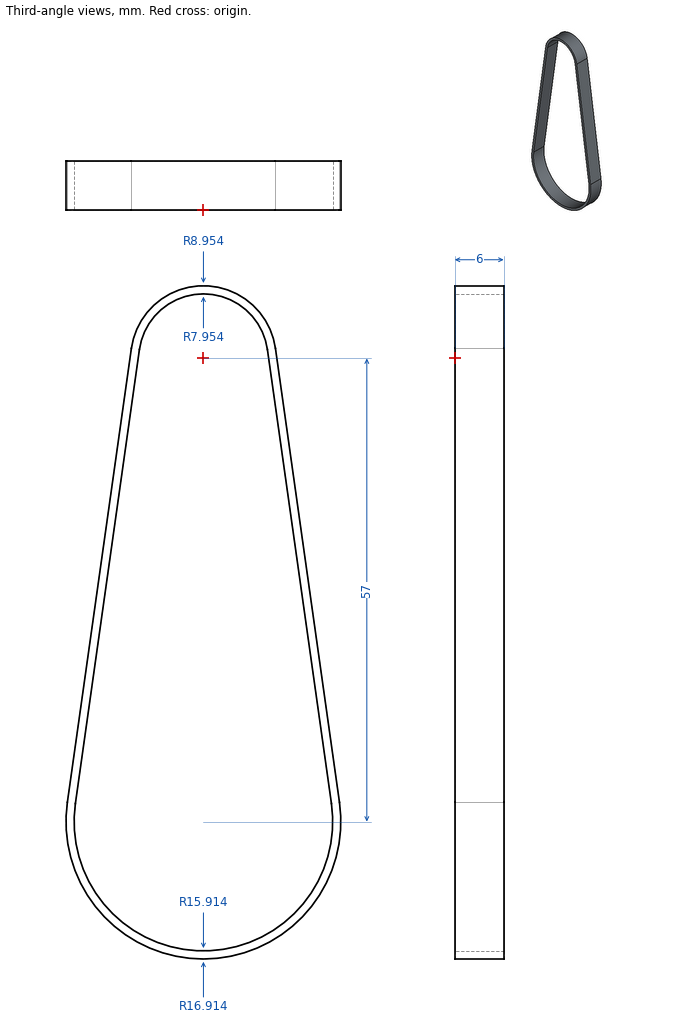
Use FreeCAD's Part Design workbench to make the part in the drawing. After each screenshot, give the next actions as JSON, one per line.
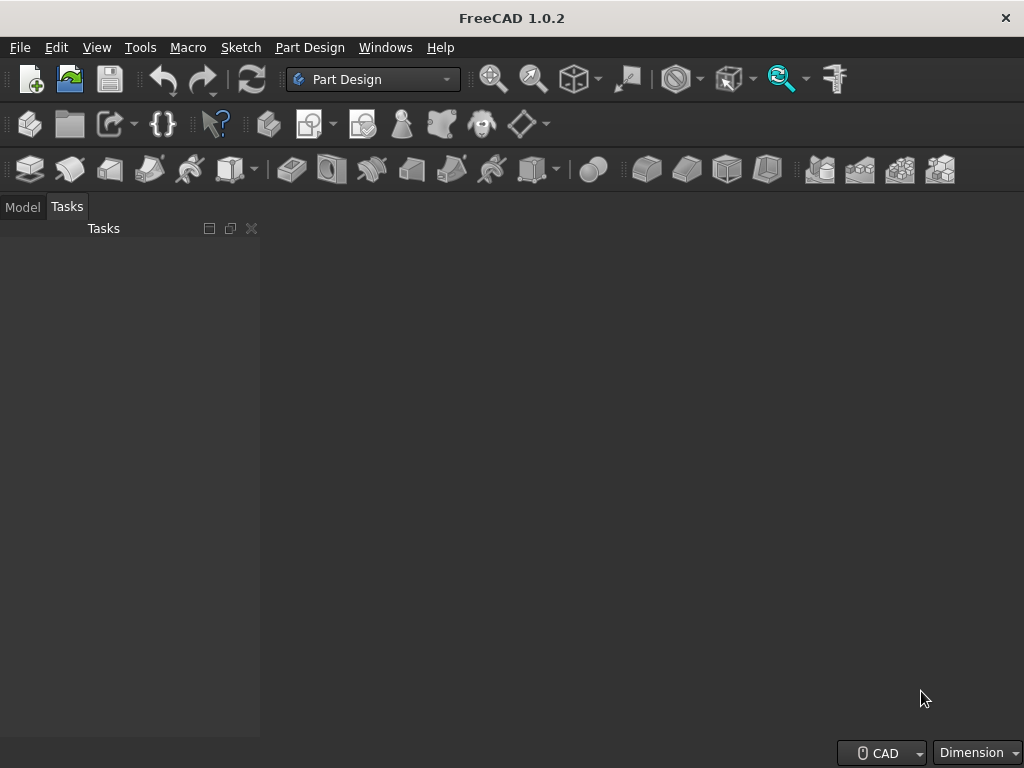
{"action": "left_click", "coordinate": [30, 80]}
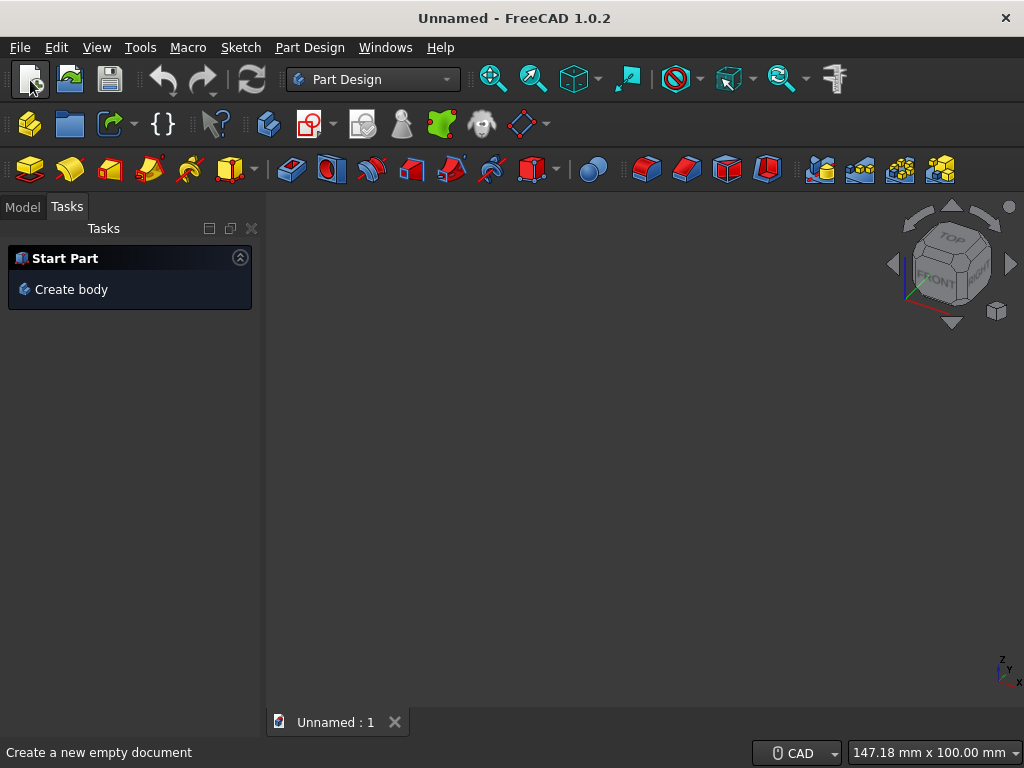
{"action": "left_click", "coordinate": [310, 124]}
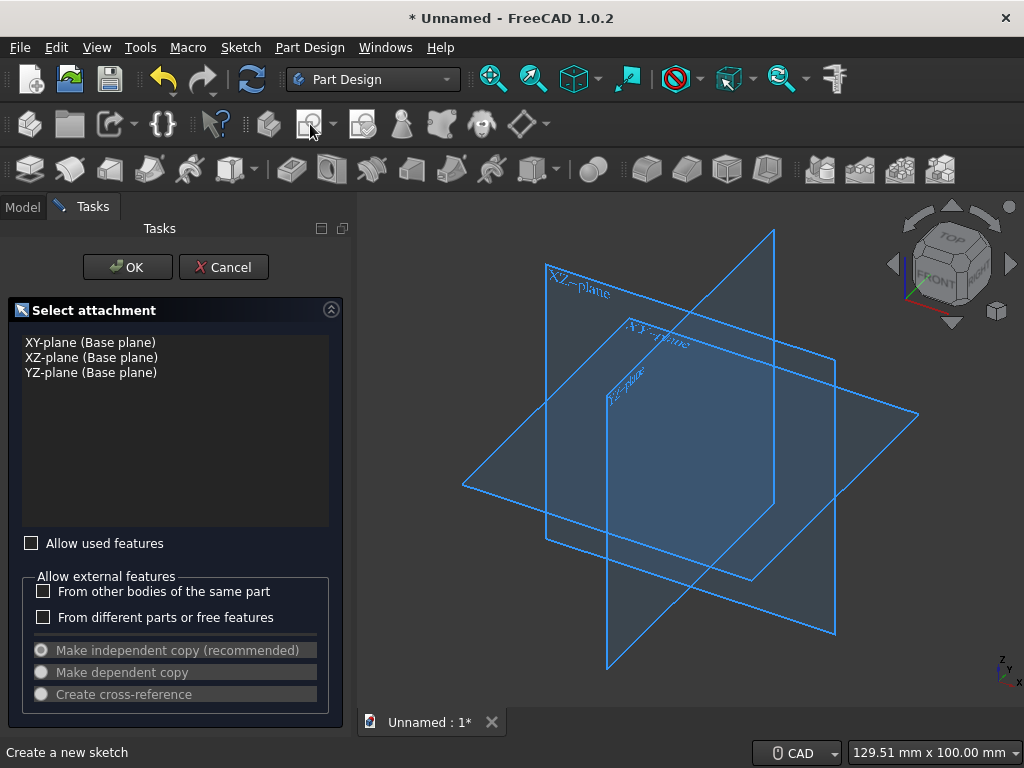
{"action": "left_click", "coordinate": [82, 358]}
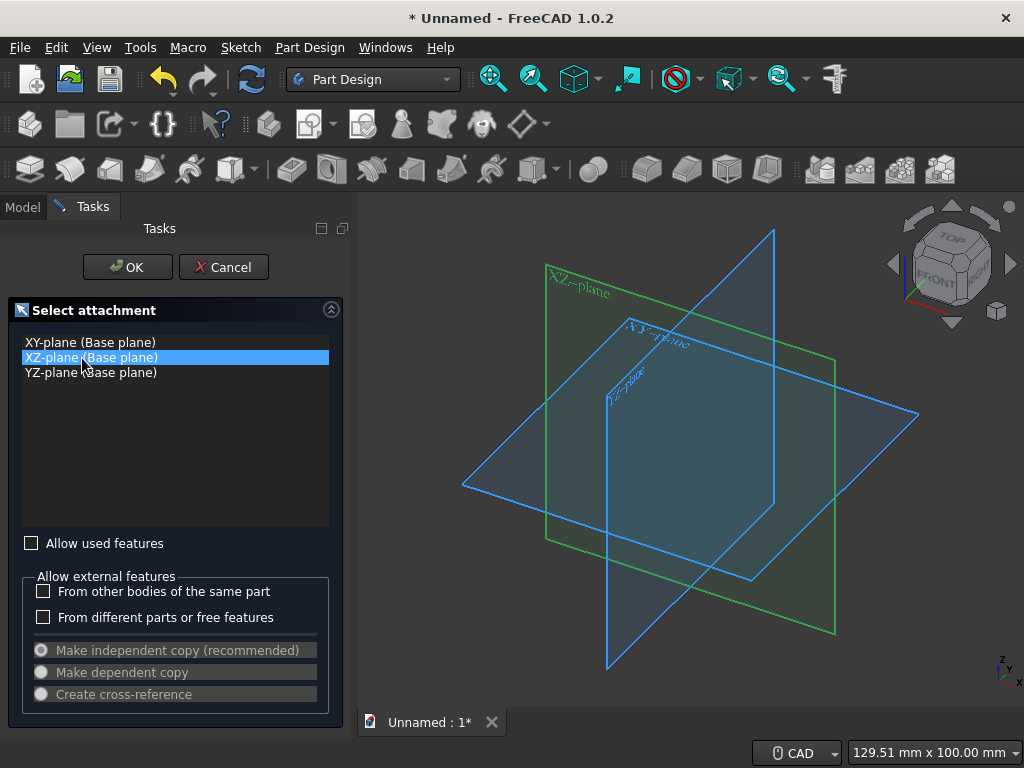
{"action": "left_click", "coordinate": [128, 267]}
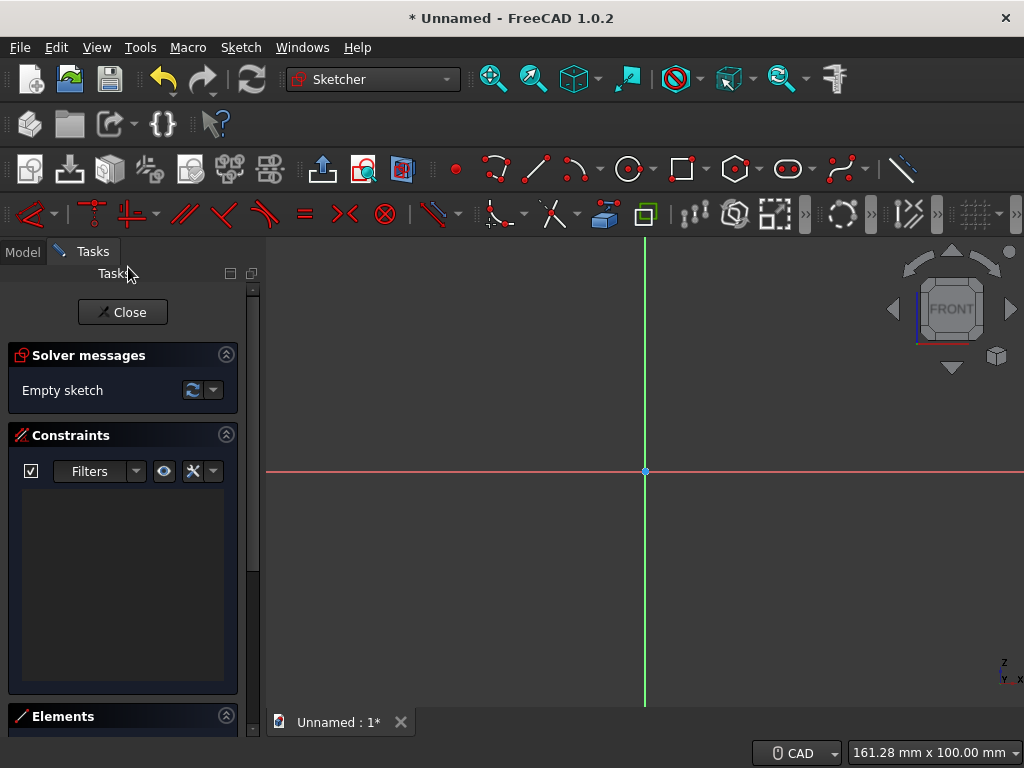
{"action": "scroll", "coordinate": [437, 265], "scroll_direction": "down", "scroll_amount": 2}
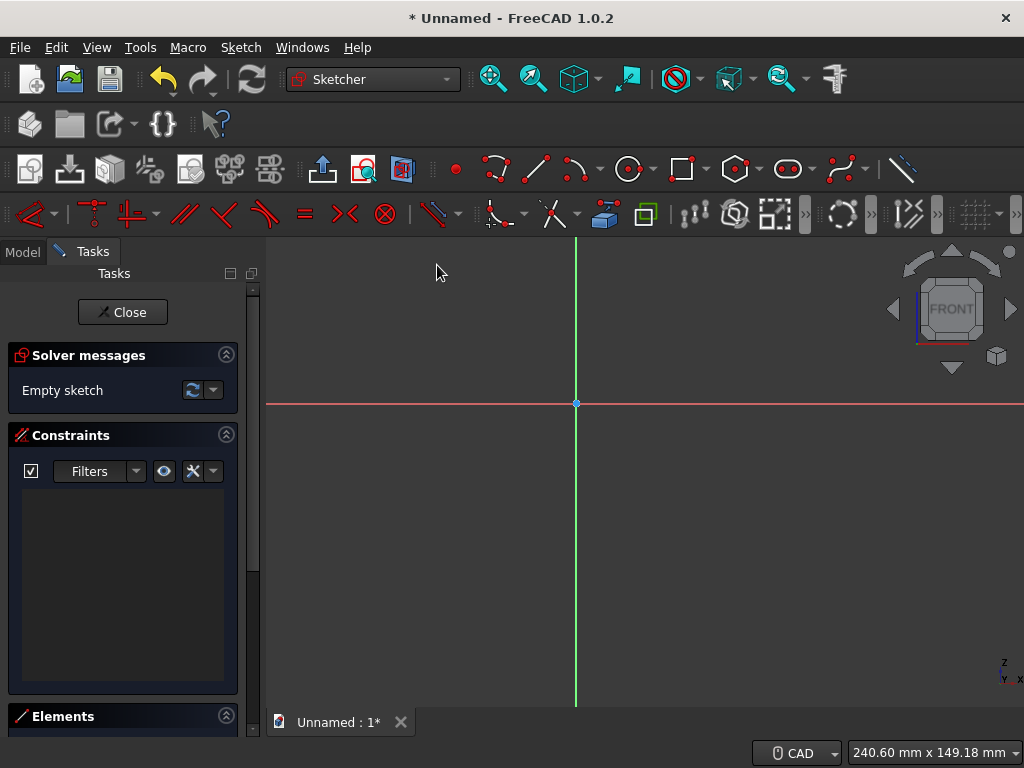
{"action": "left_click", "coordinate": [536, 170]}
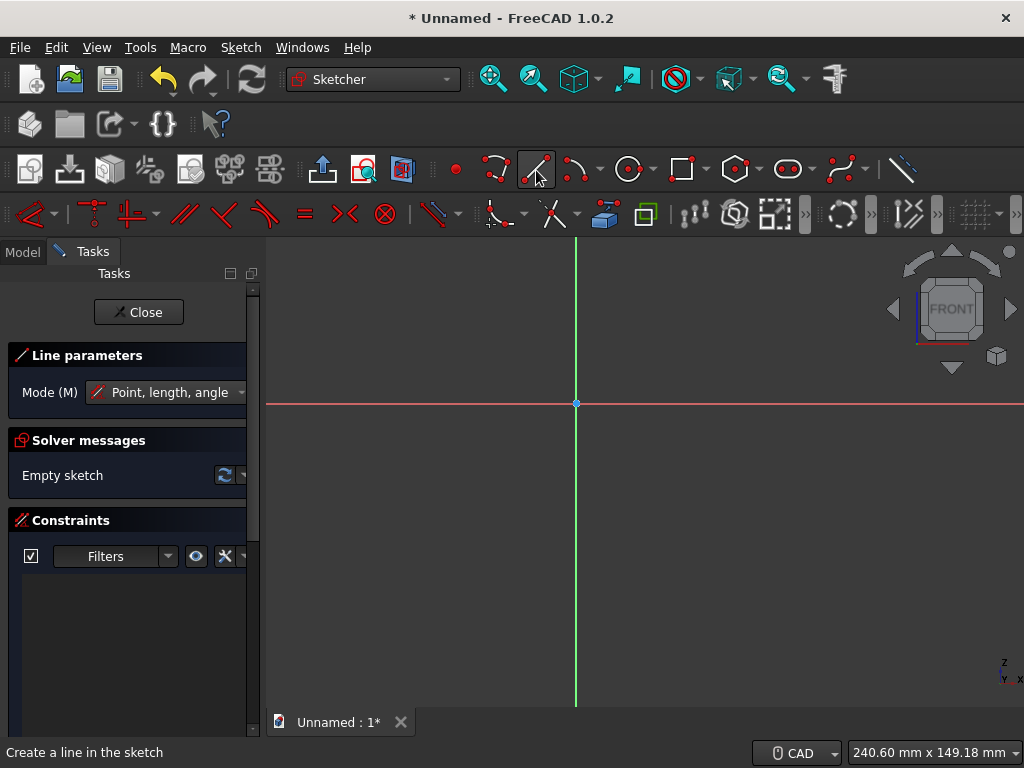
{"action": "left_click", "coordinate": [524, 576]}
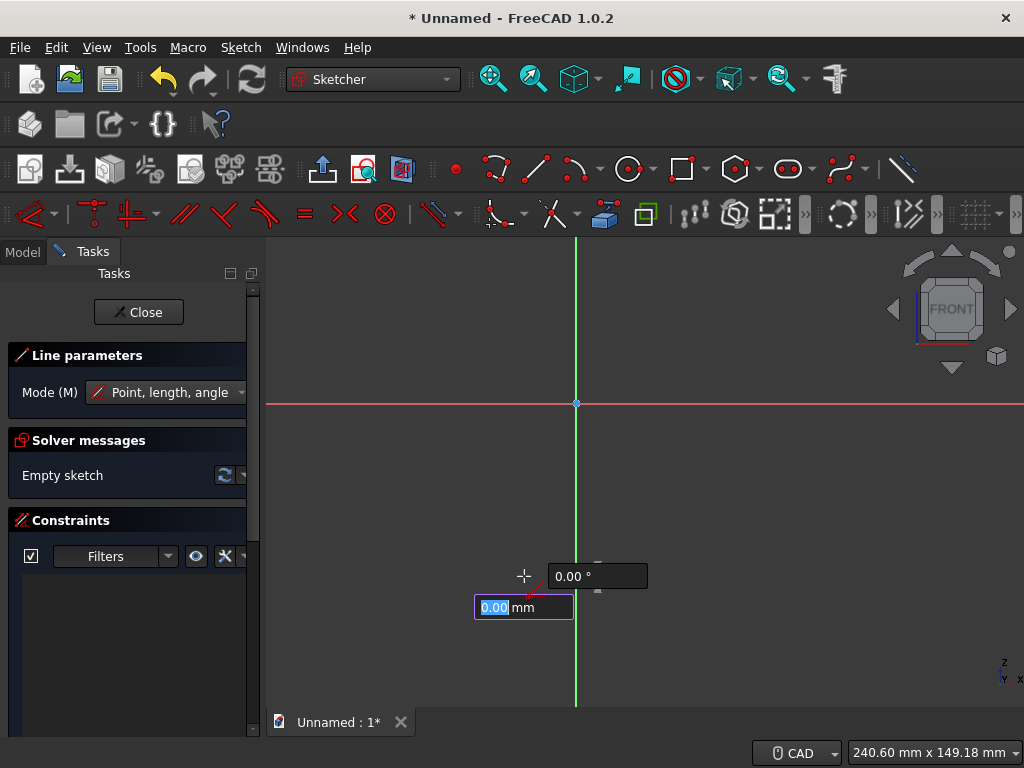
{"action": "scroll", "coordinate": [549, 400], "scroll_direction": "up", "scroll_amount": 7}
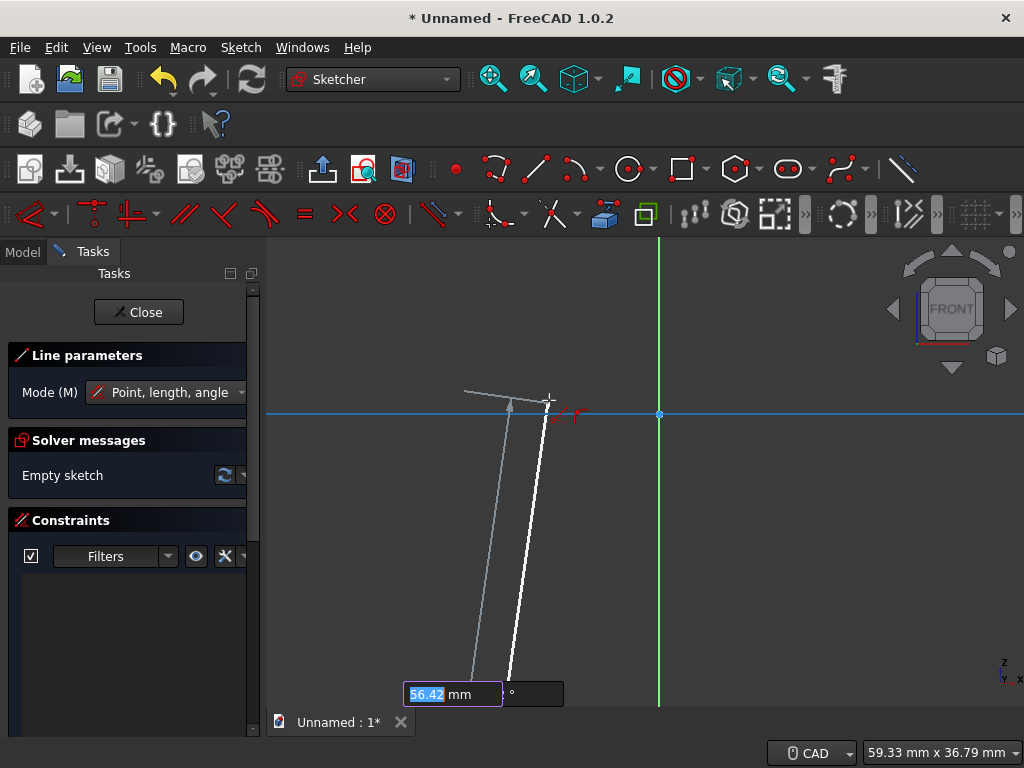
{"action": "left_click", "coordinate": [546, 398]}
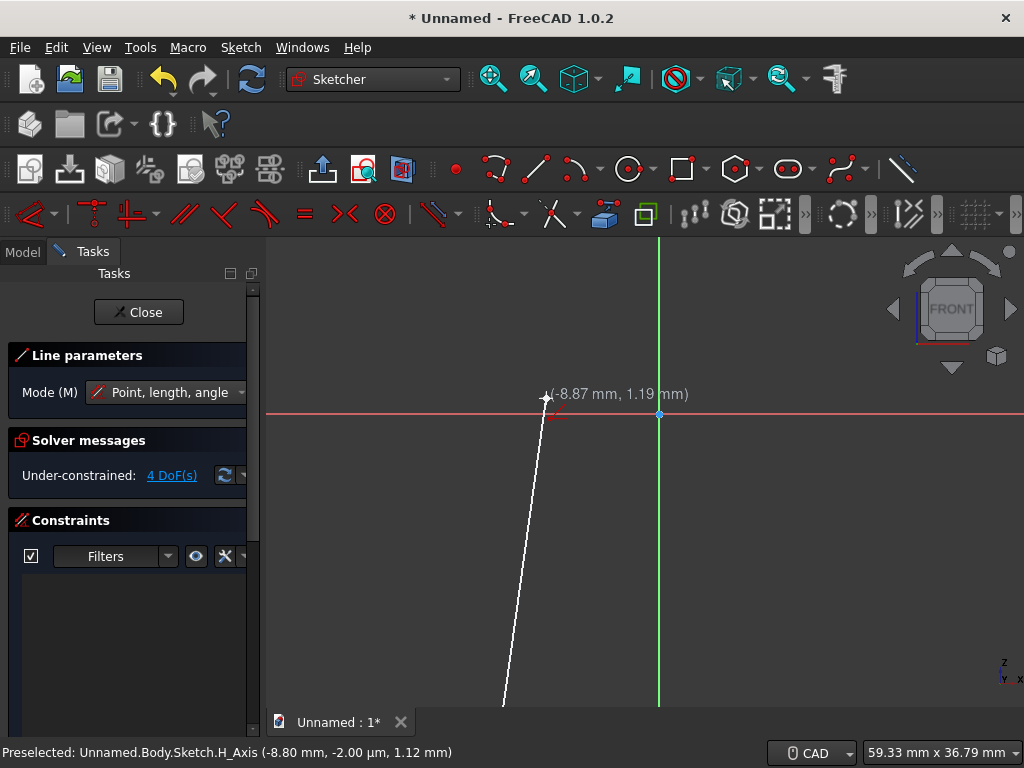
{"action": "left_click", "coordinate": [773, 398]}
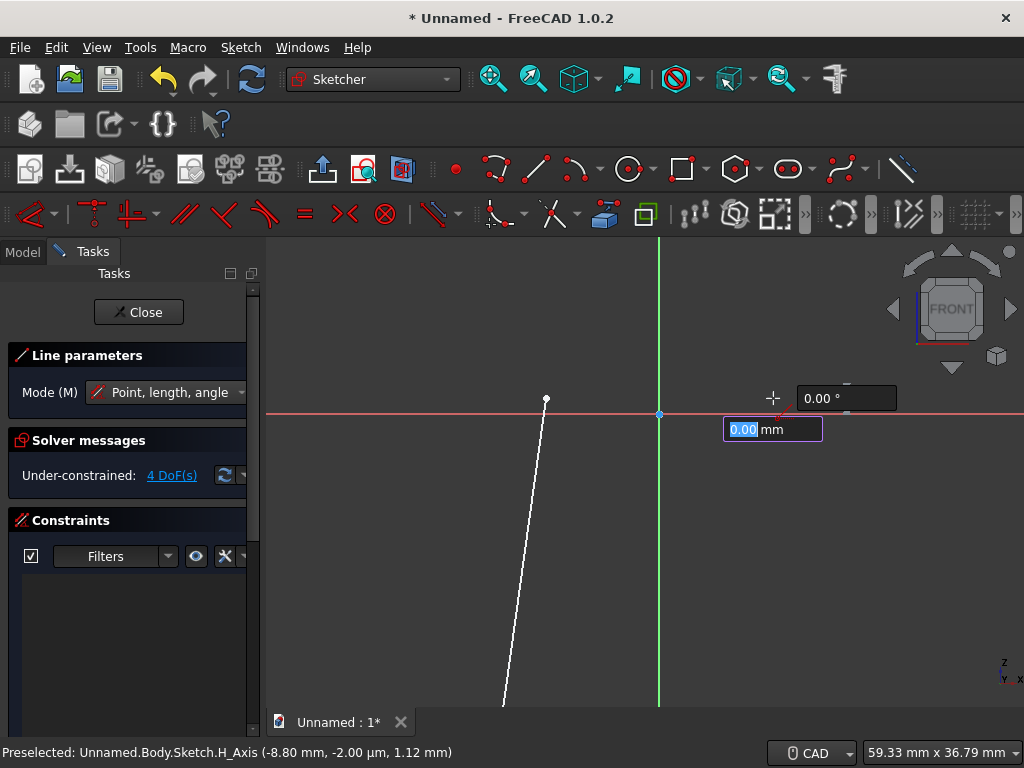
{"action": "scroll", "coordinate": [541, 318], "scroll_direction": "down", "scroll_amount": 6}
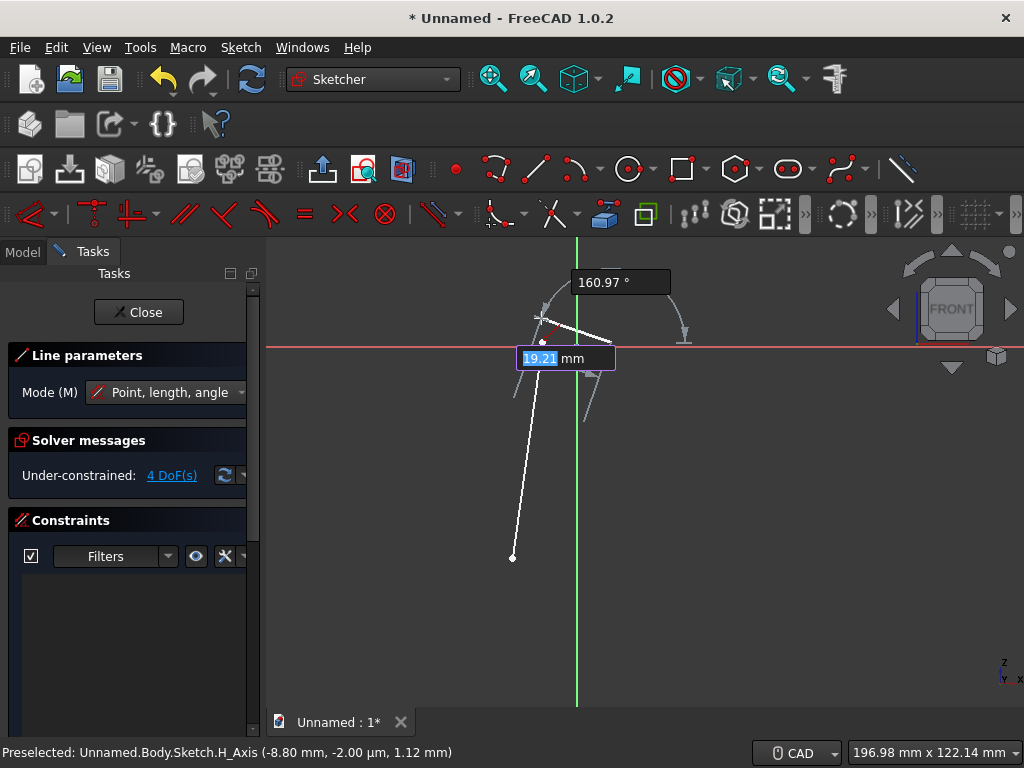
{"action": "left_click", "coordinate": [641, 557]}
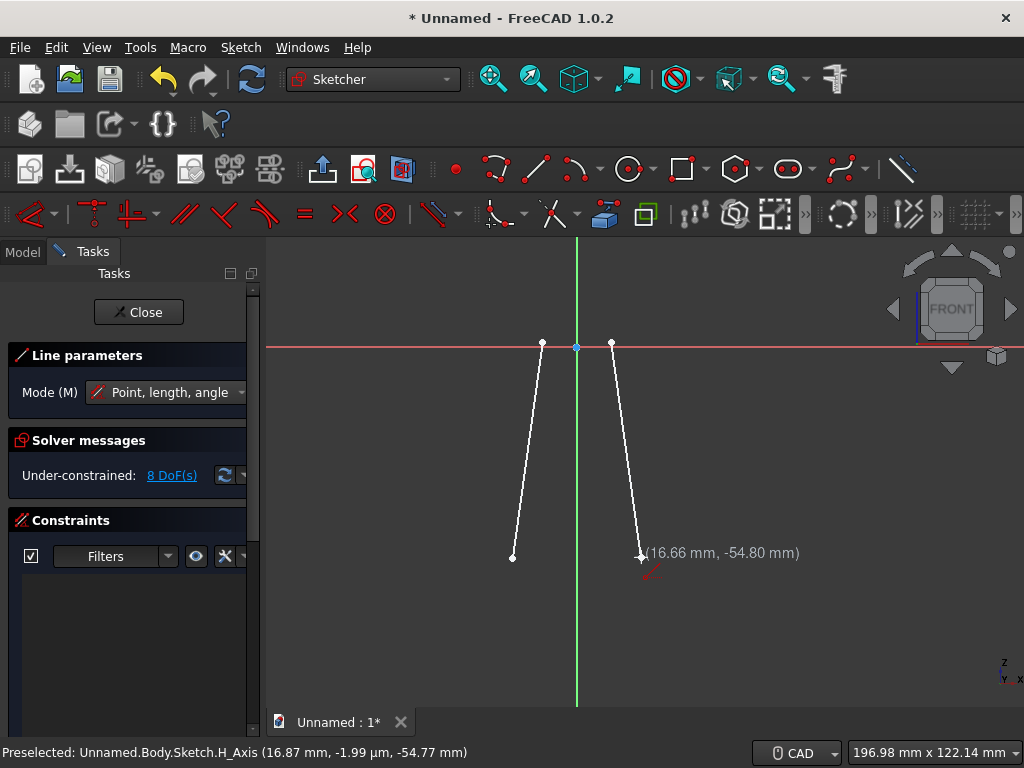
{"action": "left_click", "coordinate": [602, 170]}